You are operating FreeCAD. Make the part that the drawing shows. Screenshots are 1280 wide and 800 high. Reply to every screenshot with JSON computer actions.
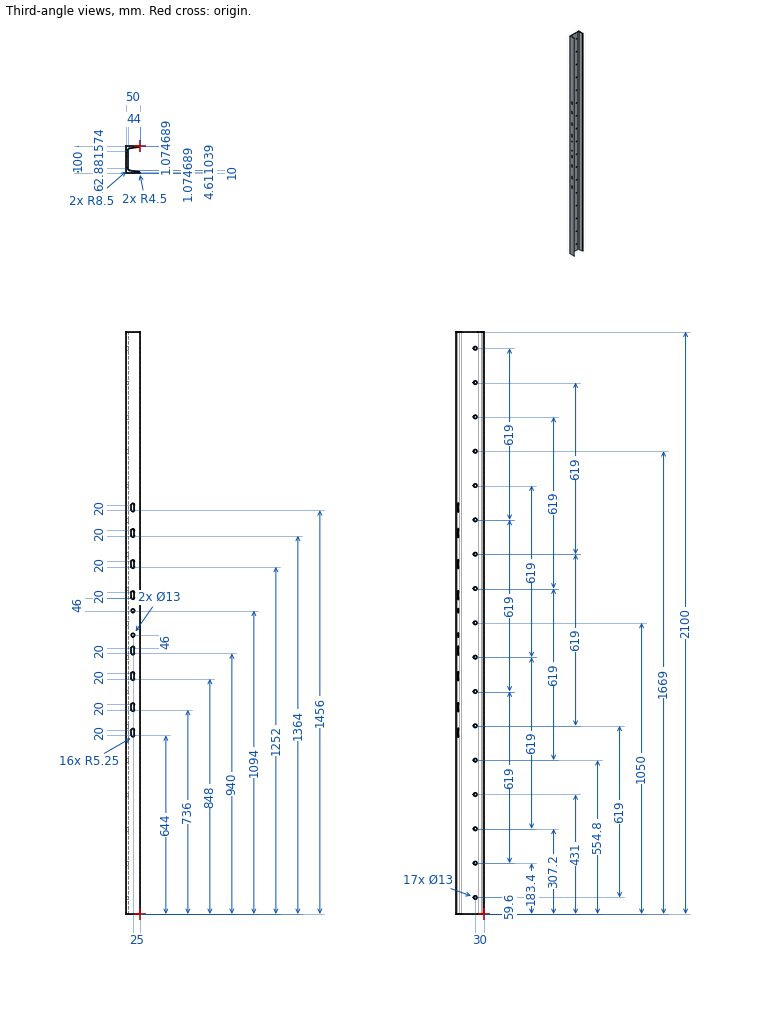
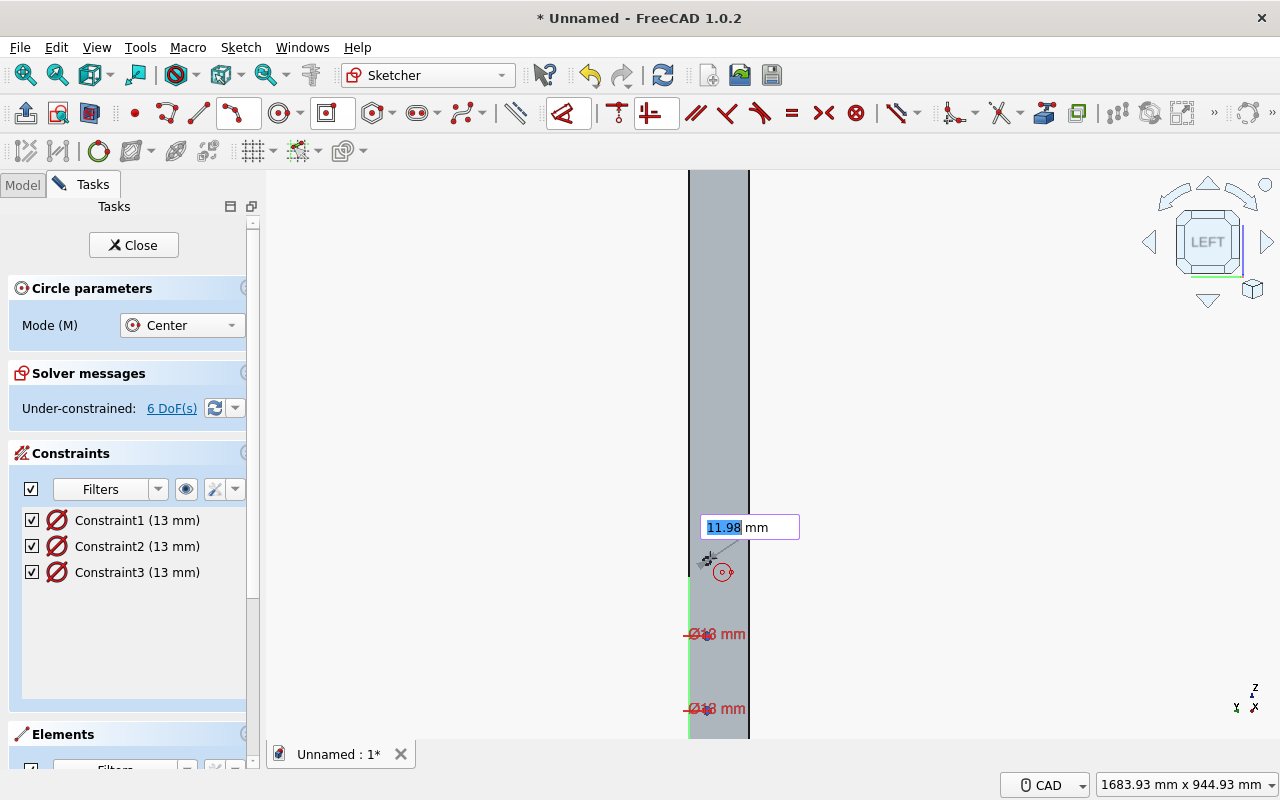
{"action": "type", "text": "13"}
{"action": "key", "text": "Return"}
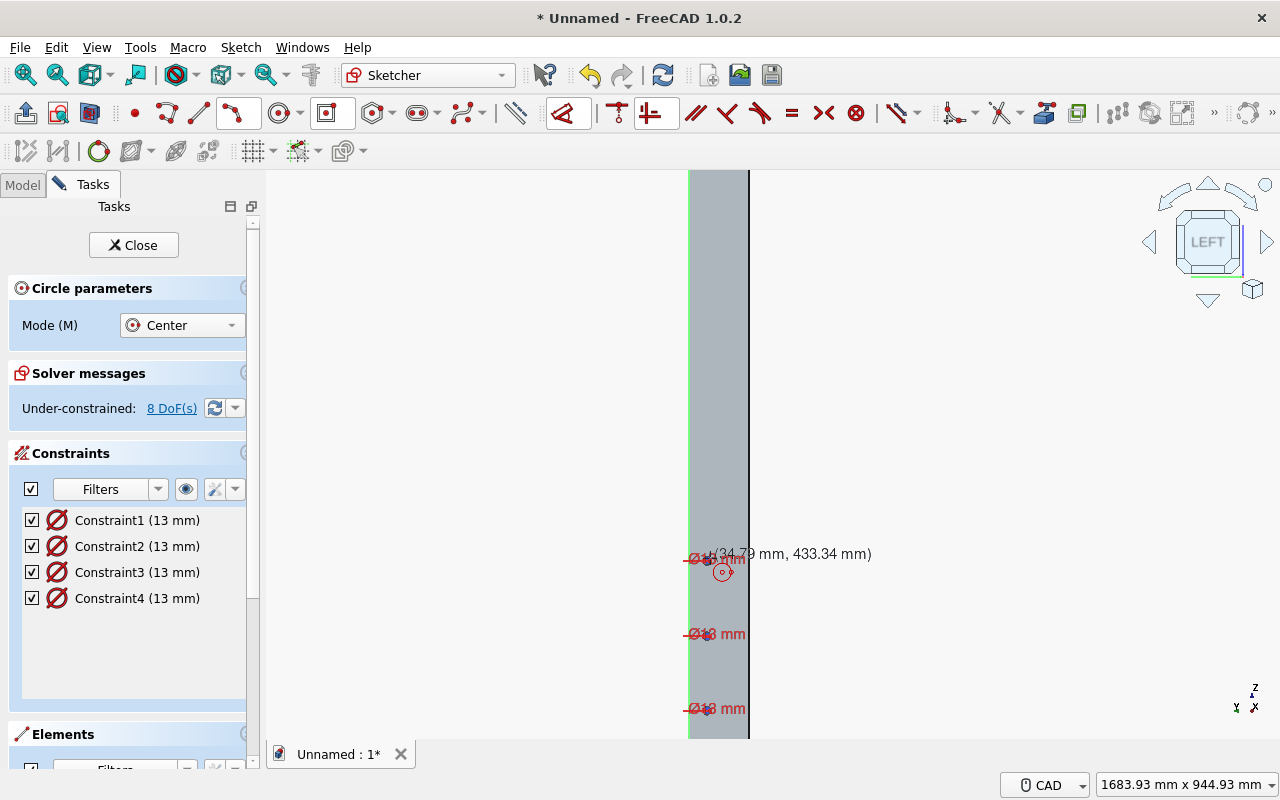
{"action": "scroll", "coordinate": [707, 486], "scroll_direction": "up", "scroll_amount": 9}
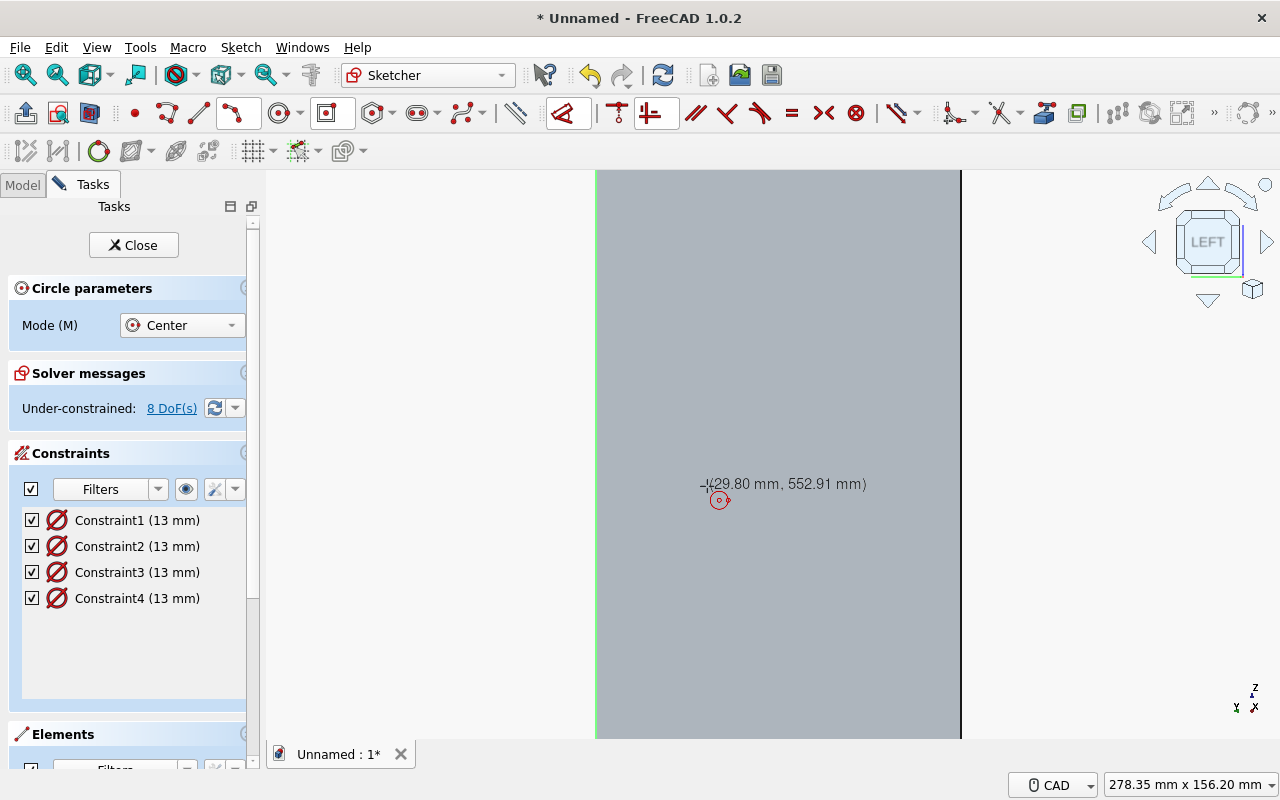
{"action": "scroll", "coordinate": [707, 542], "scroll_direction": "down", "scroll_amount": 15}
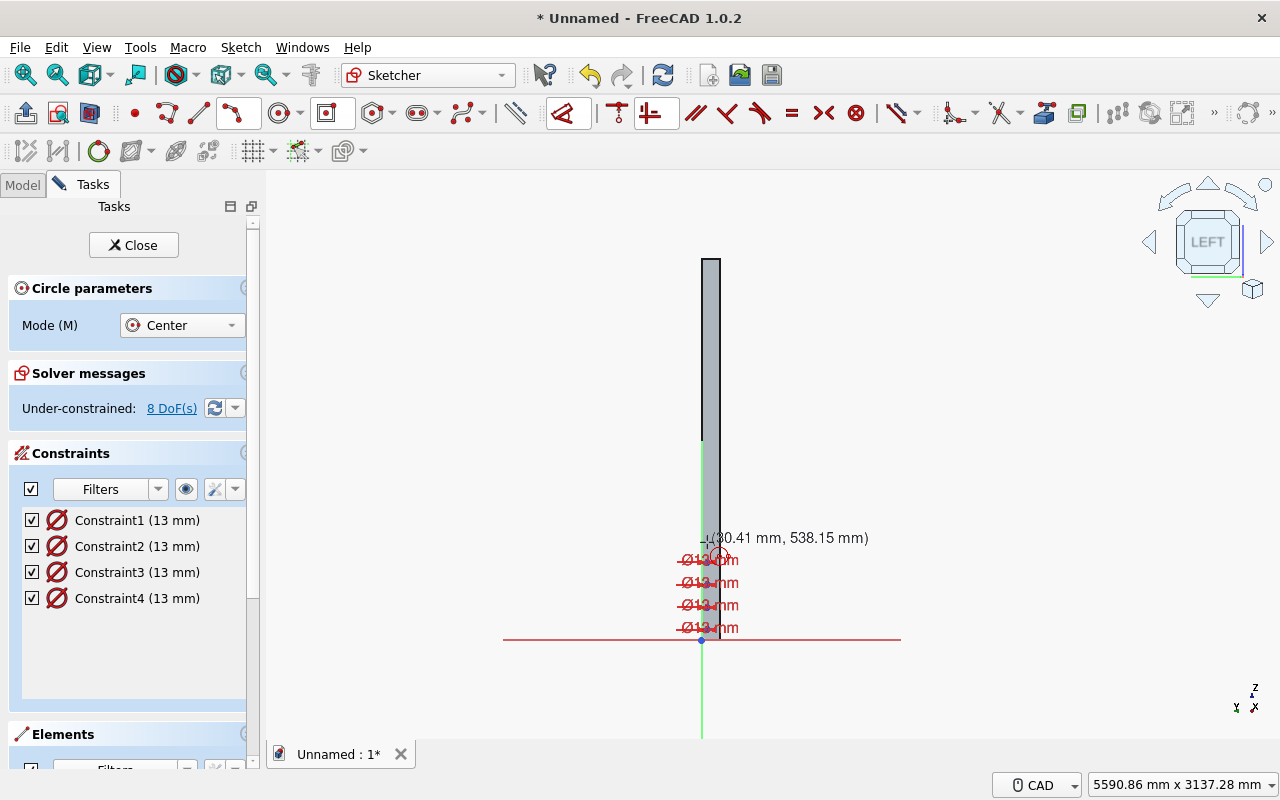
{"action": "scroll", "coordinate": [707, 540], "scroll_direction": "up", "scroll_amount": 6}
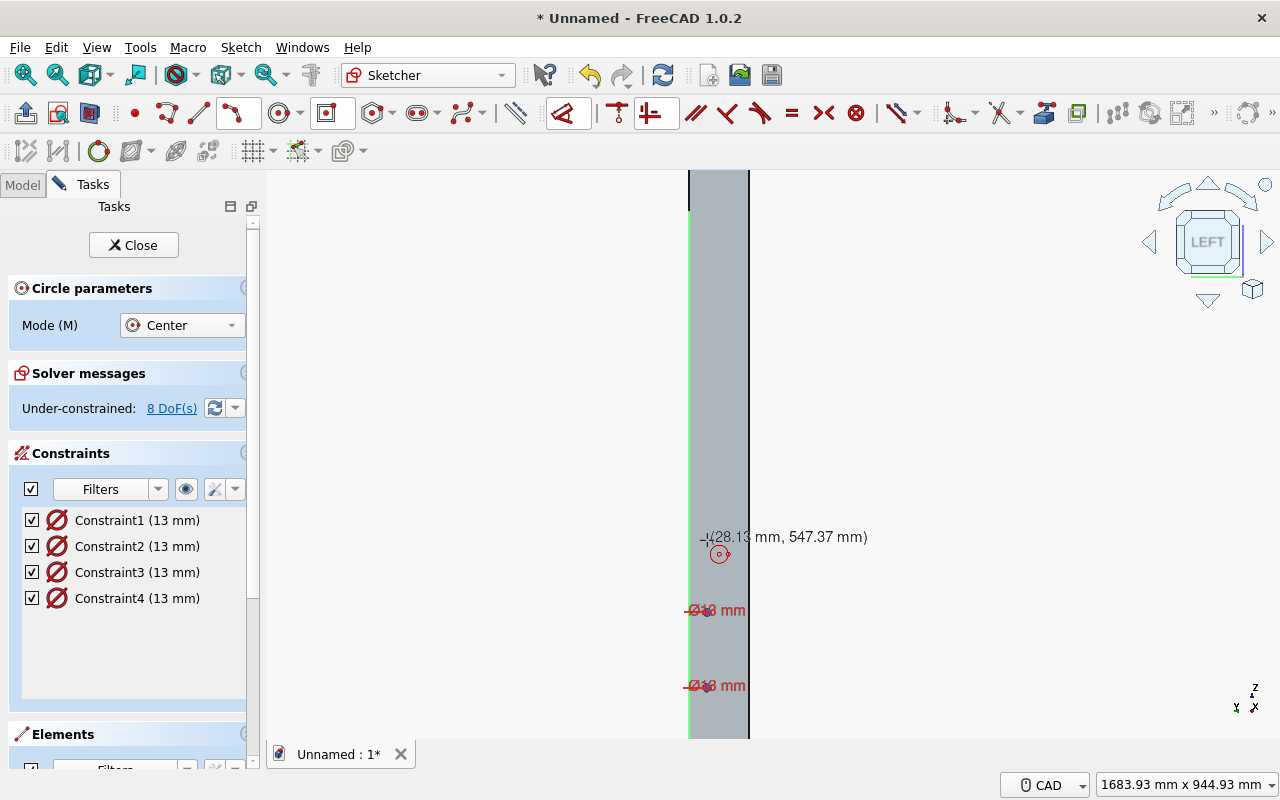
{"action": "left_click", "coordinate": [707, 537]}
{"action": "mouse_move", "coordinate": [710, 535]}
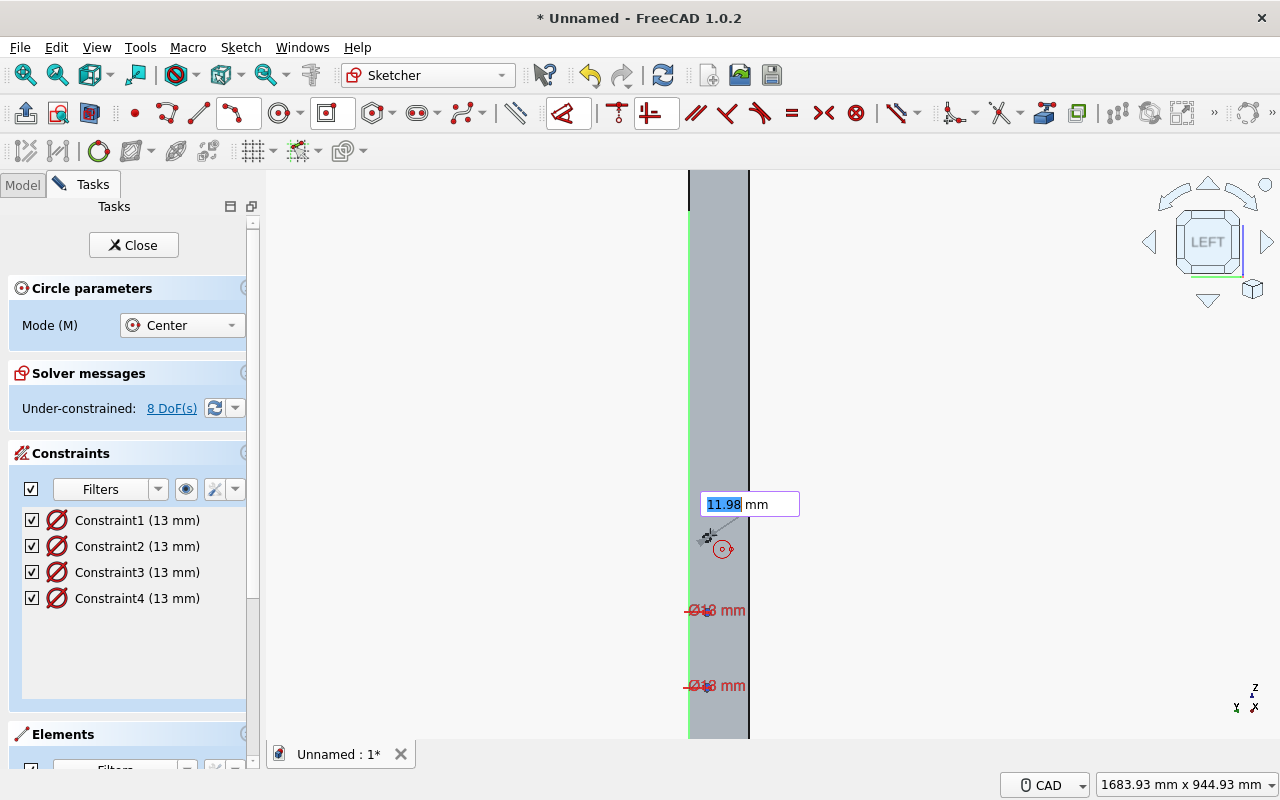
{"action": "type", "text": "13"}
{"action": "key", "text": "Return"}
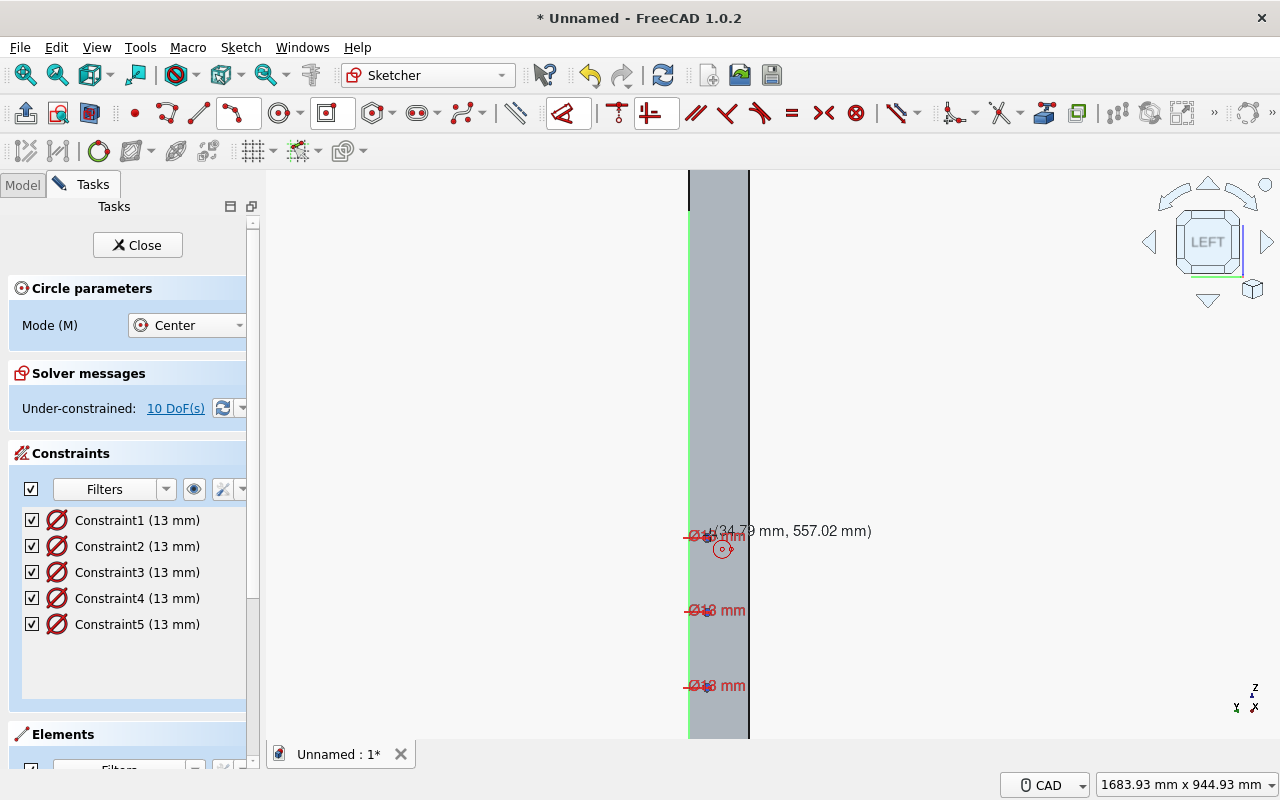
{"action": "scroll", "coordinate": [707, 463], "scroll_direction": "up", "scroll_amount": 9}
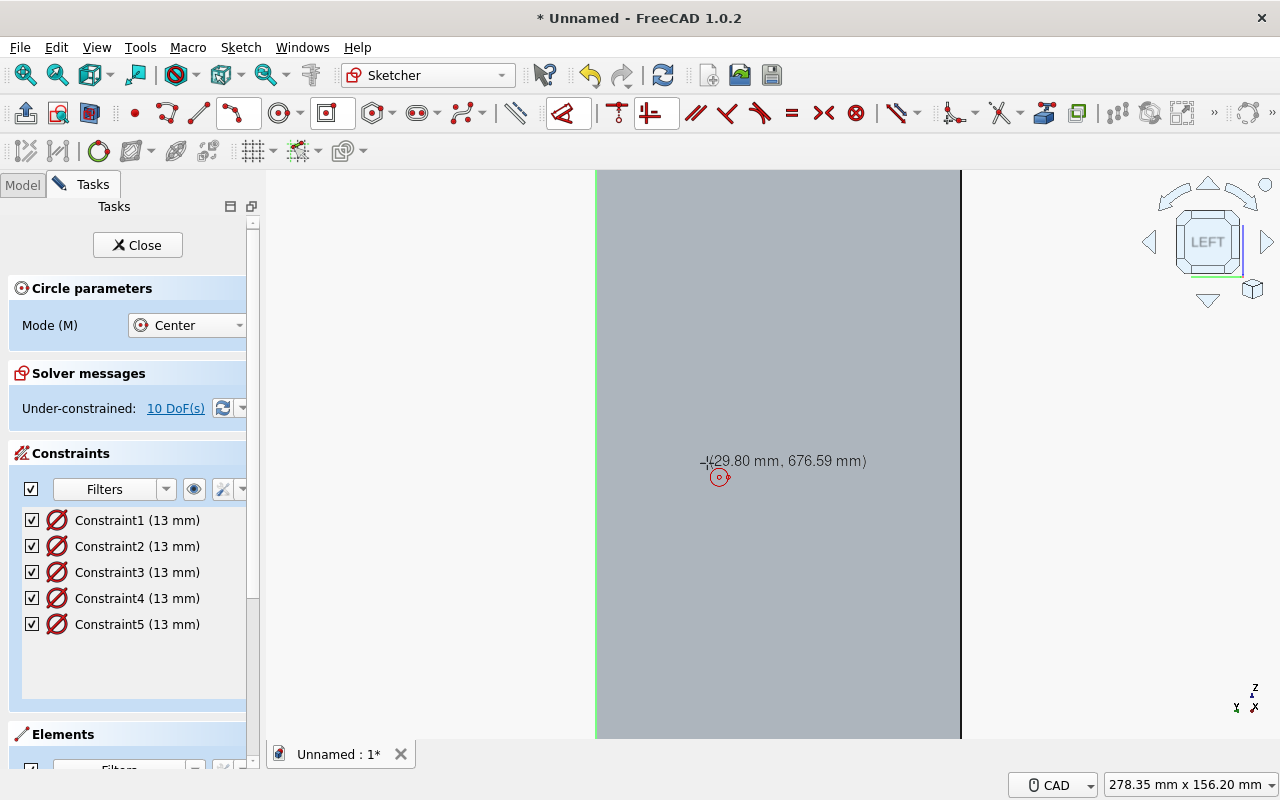
{"action": "scroll", "coordinate": [707, 520], "scroll_direction": "down", "scroll_amount": 15}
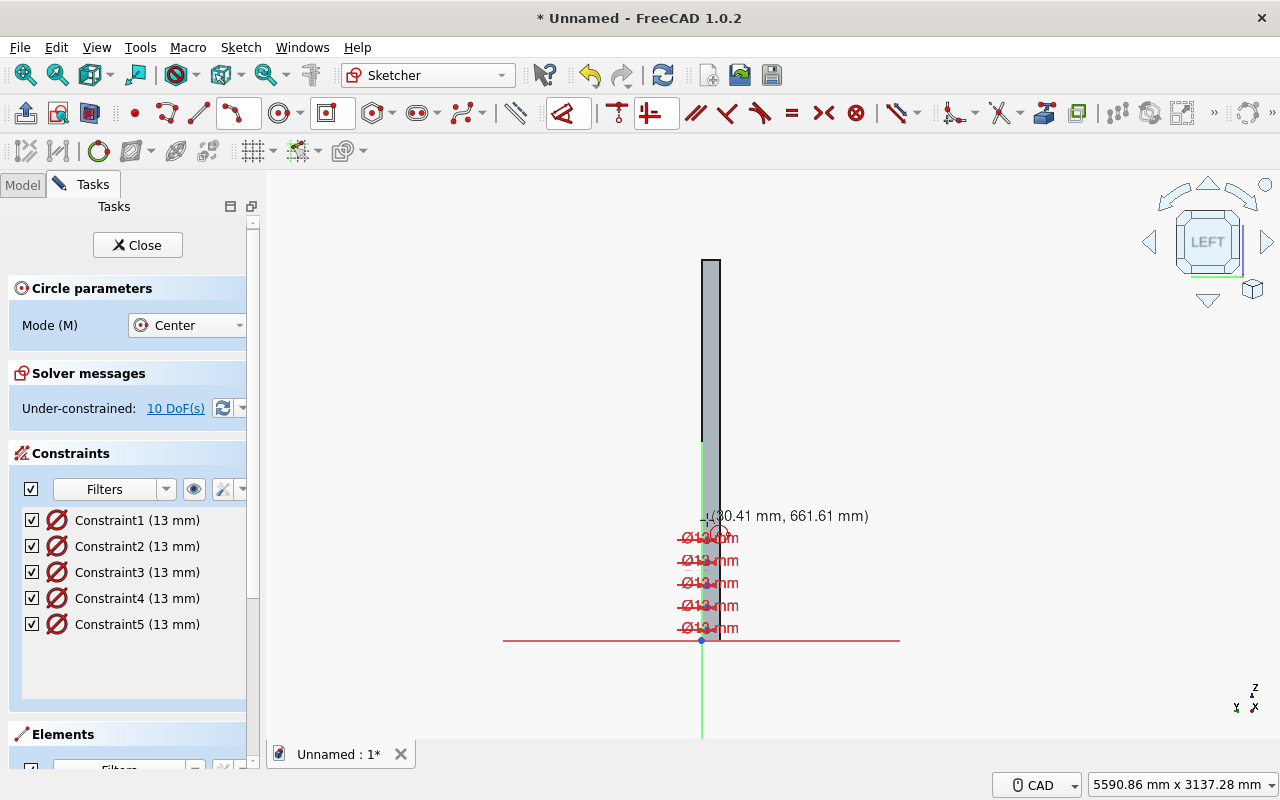
{"action": "scroll", "coordinate": [707, 518], "scroll_direction": "up", "scroll_amount": 6}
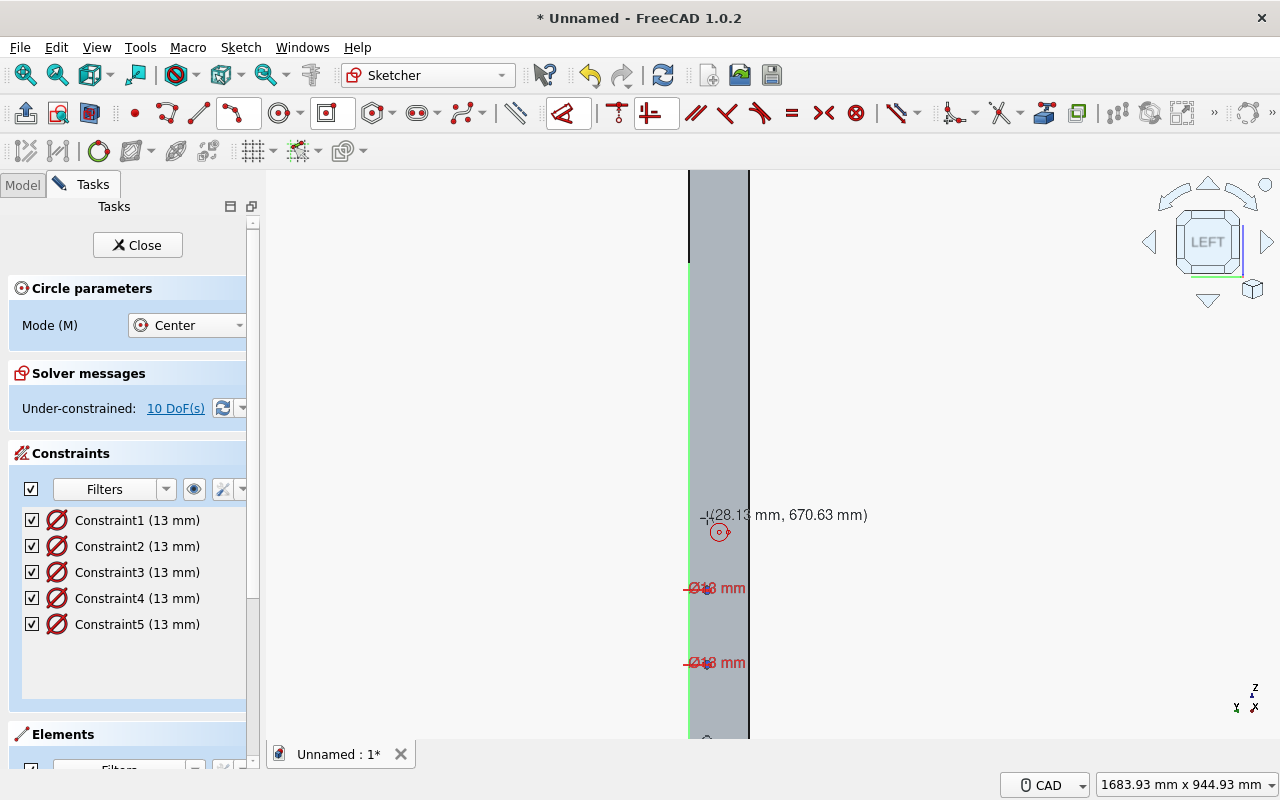
{"action": "left_click", "coordinate": [707, 515]}
{"action": "mouse_move", "coordinate": [710, 512]}